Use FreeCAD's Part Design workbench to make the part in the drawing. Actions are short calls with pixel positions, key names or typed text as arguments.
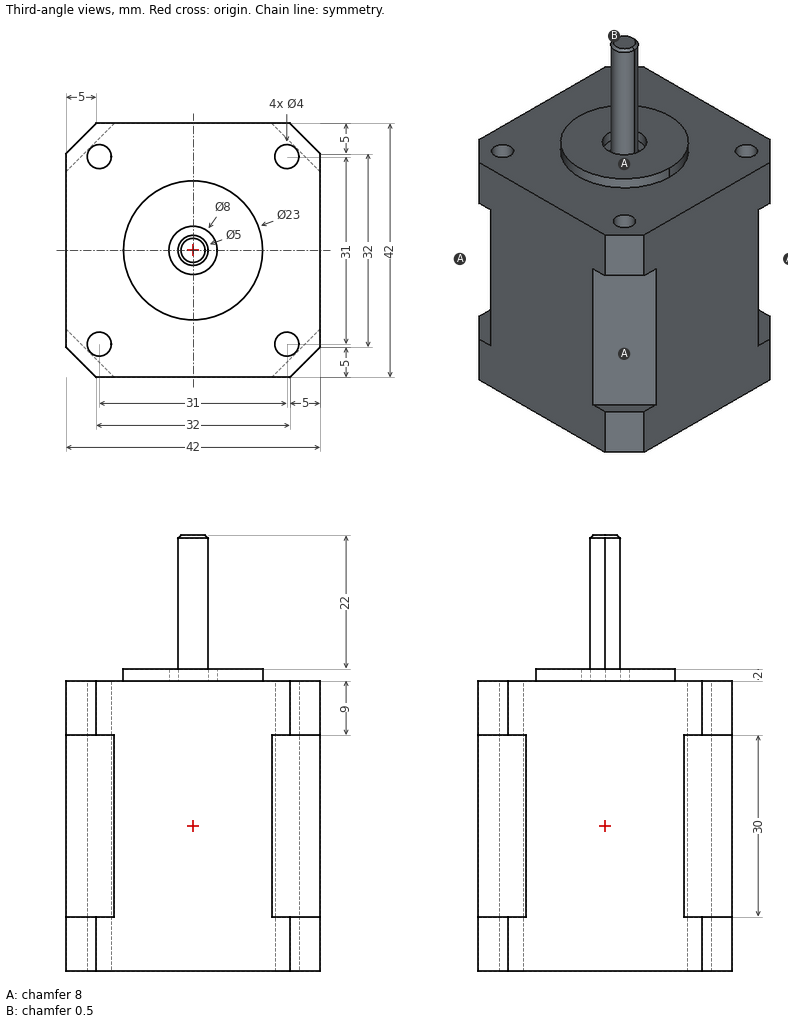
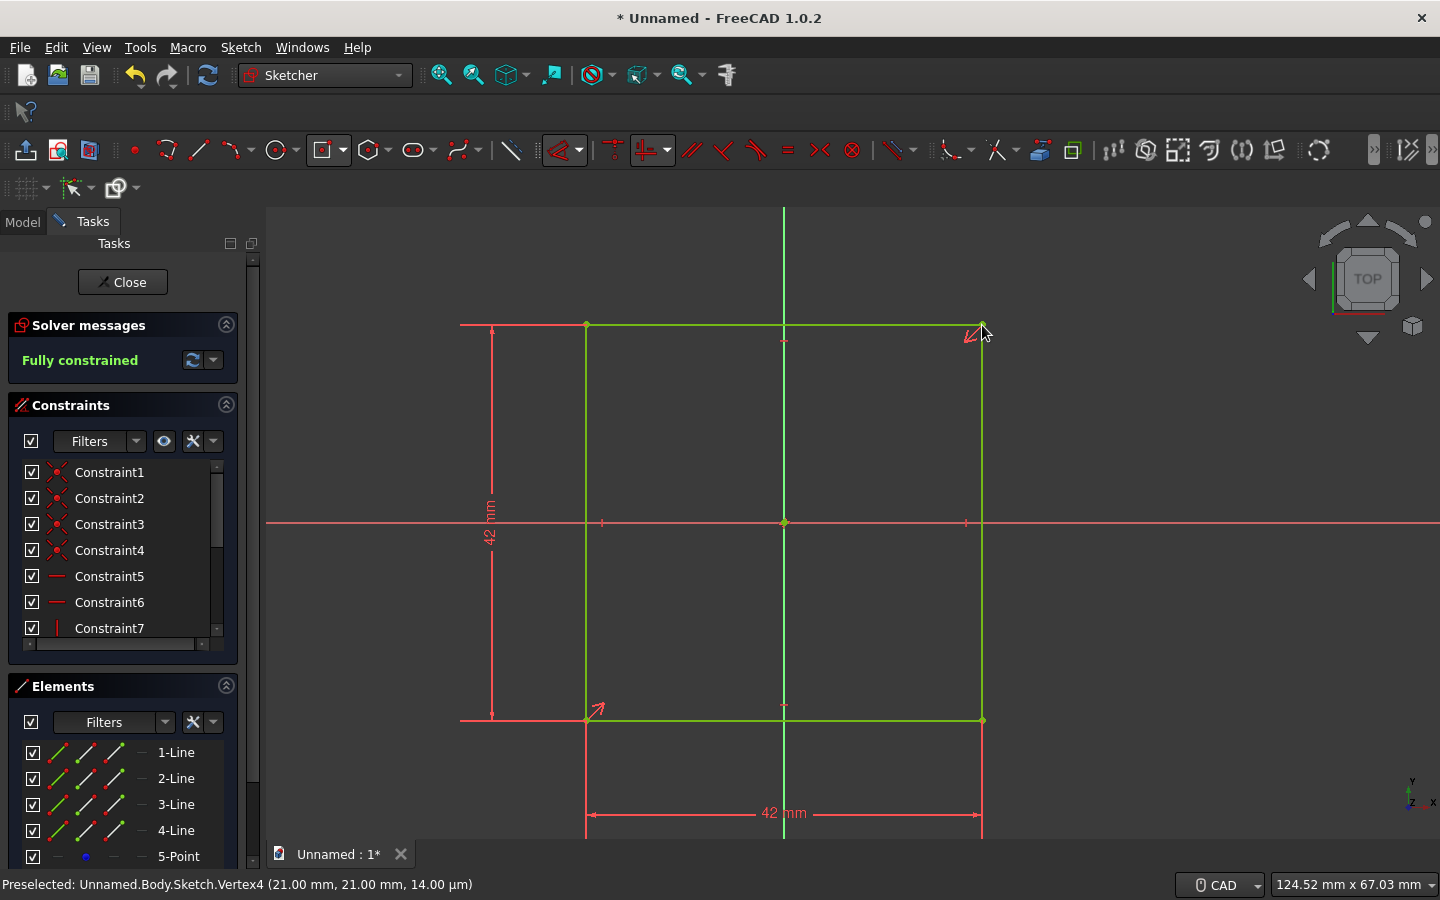
click(123, 282)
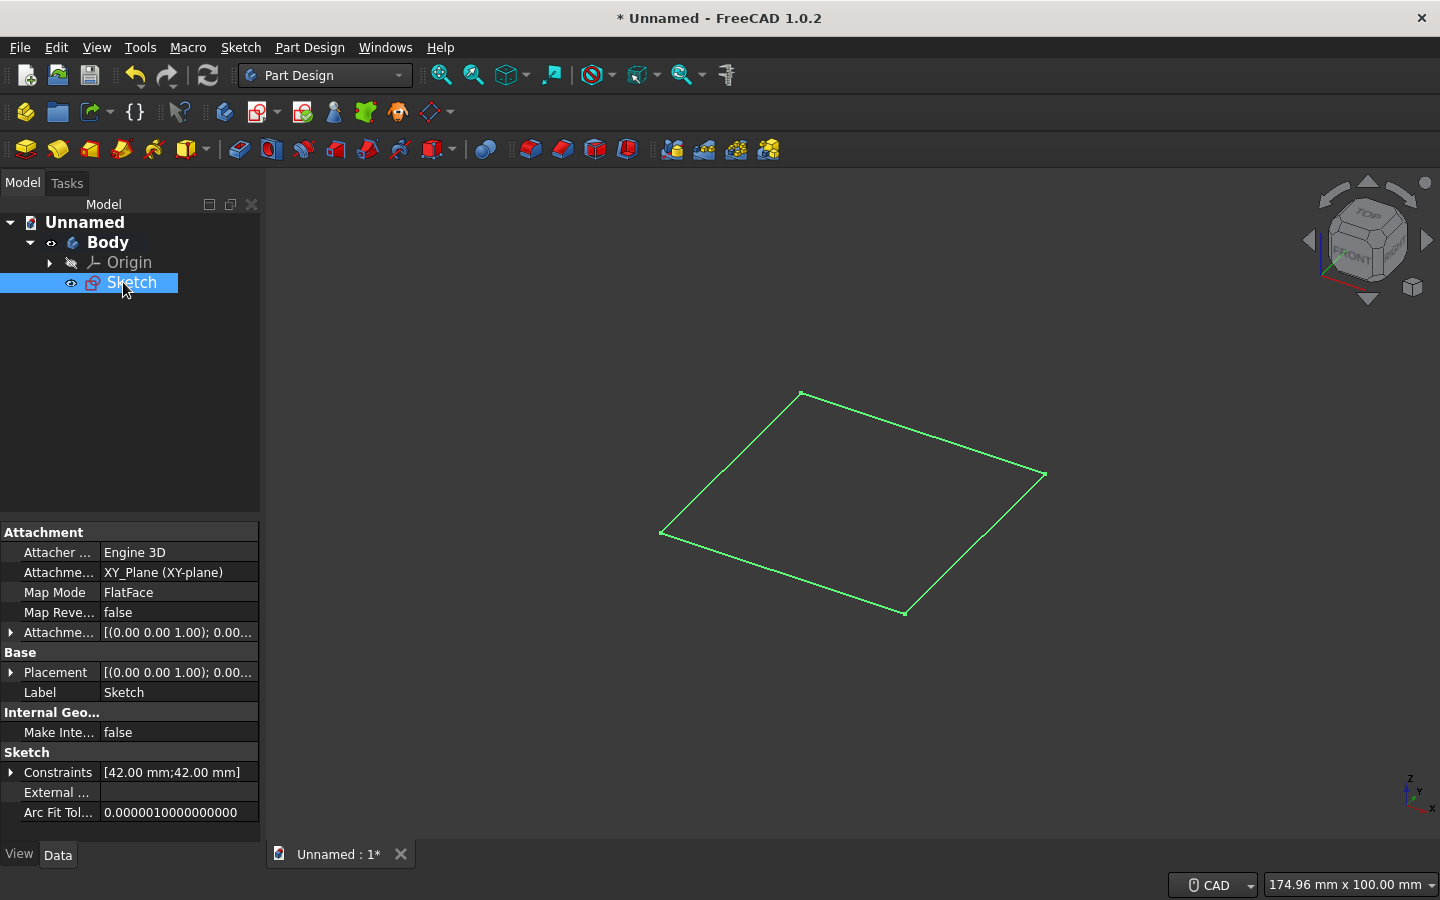
click(26, 150)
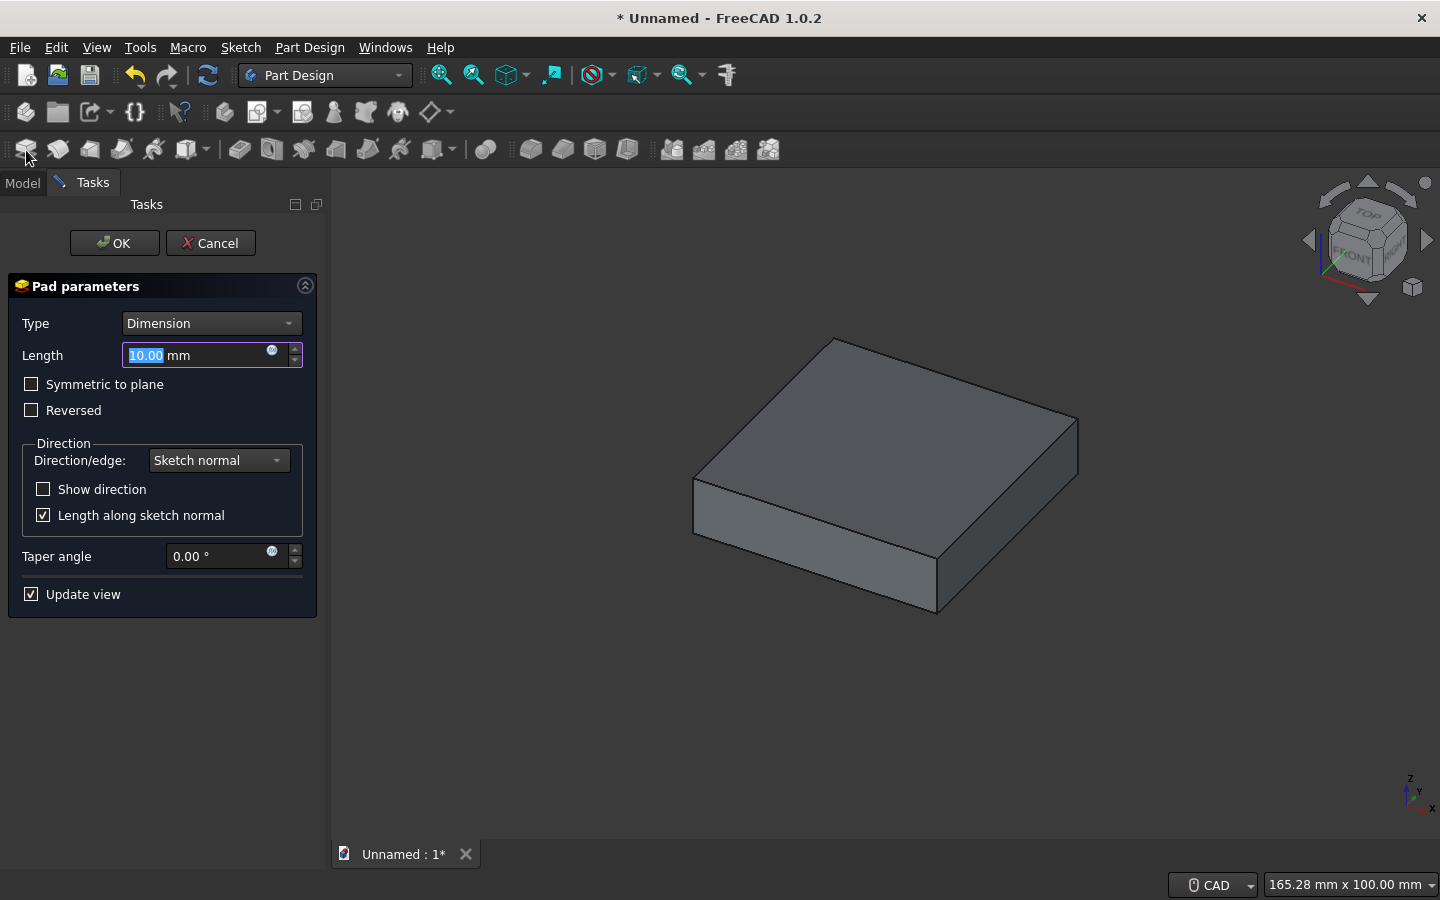
text(30)
key(Tab)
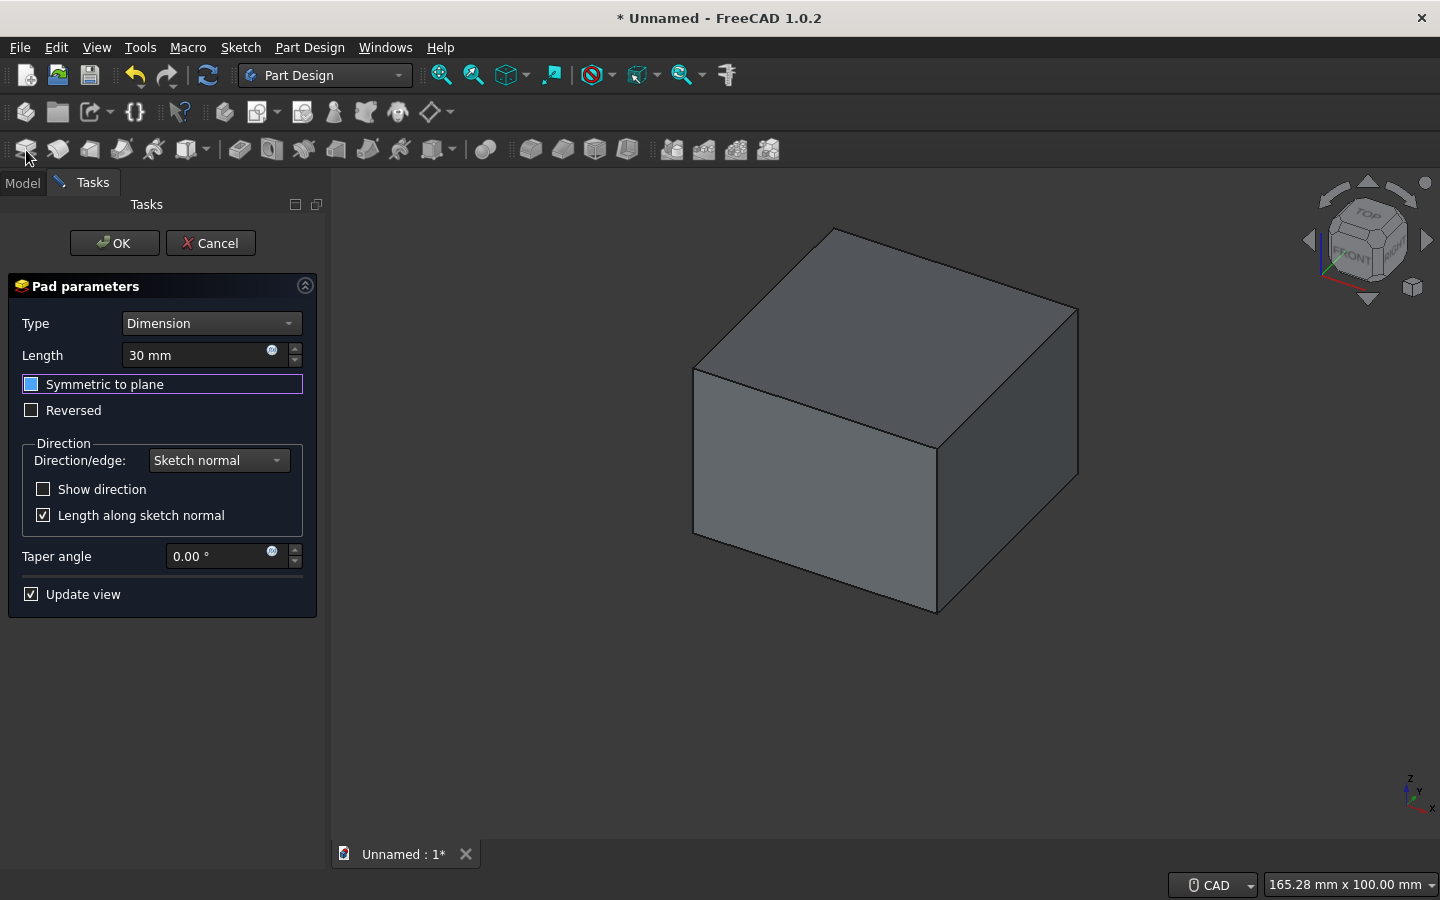
click(30, 384)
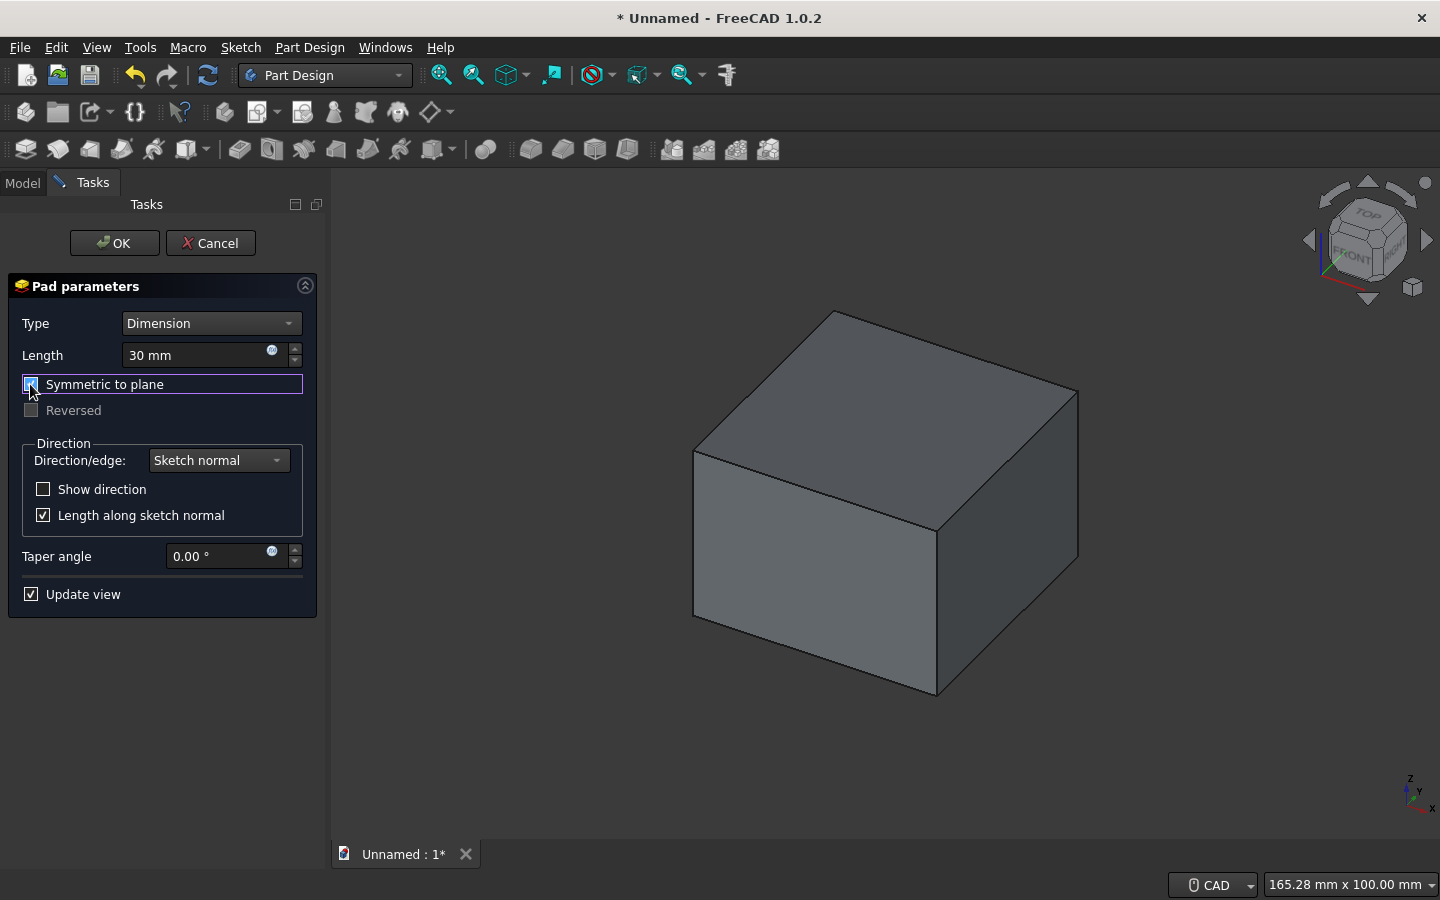
click(115, 243)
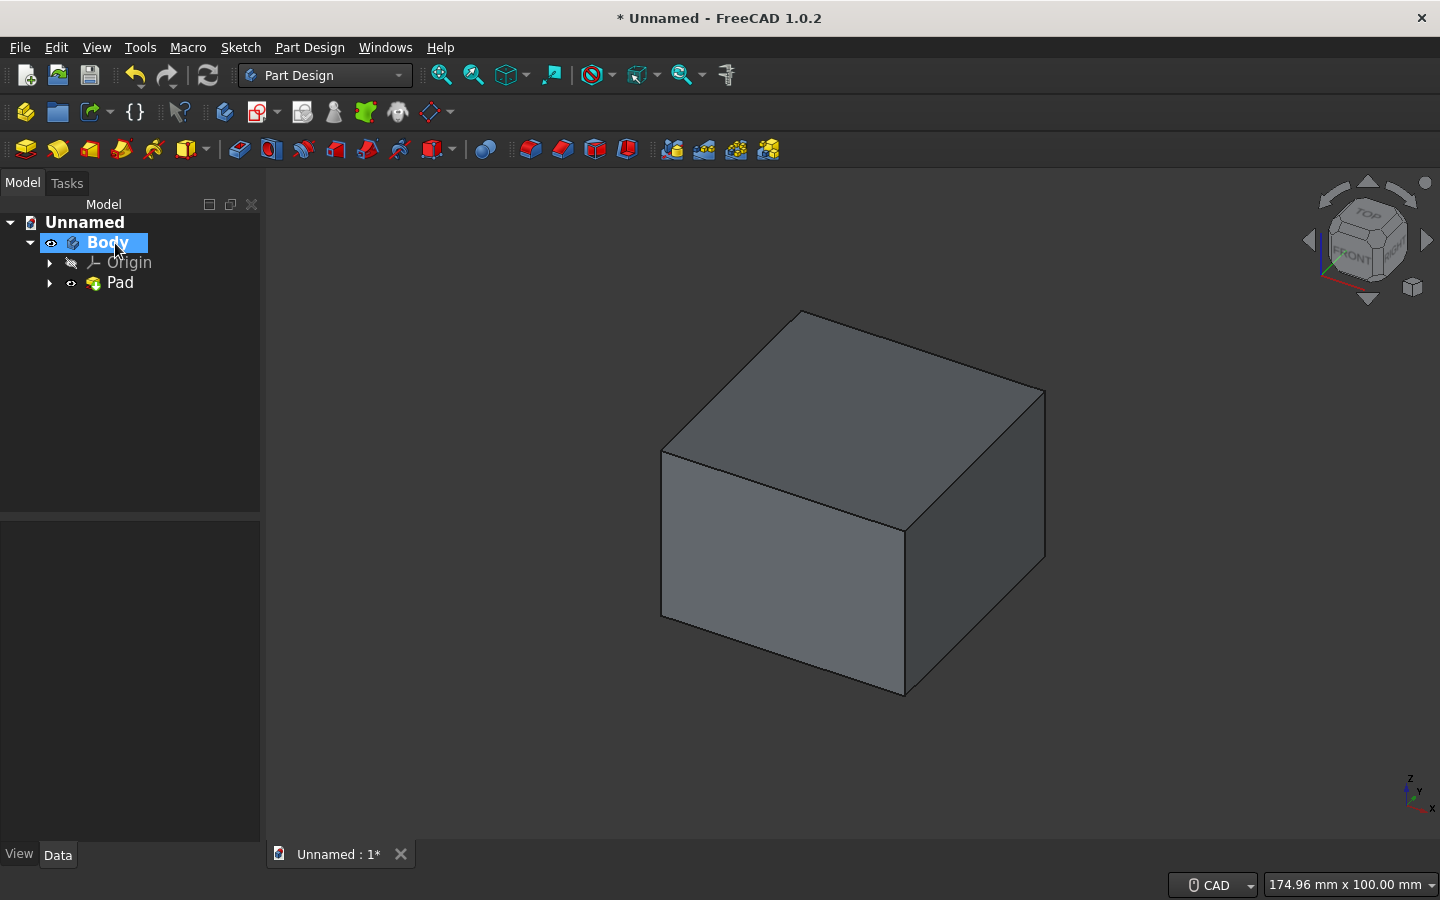
click(905, 613)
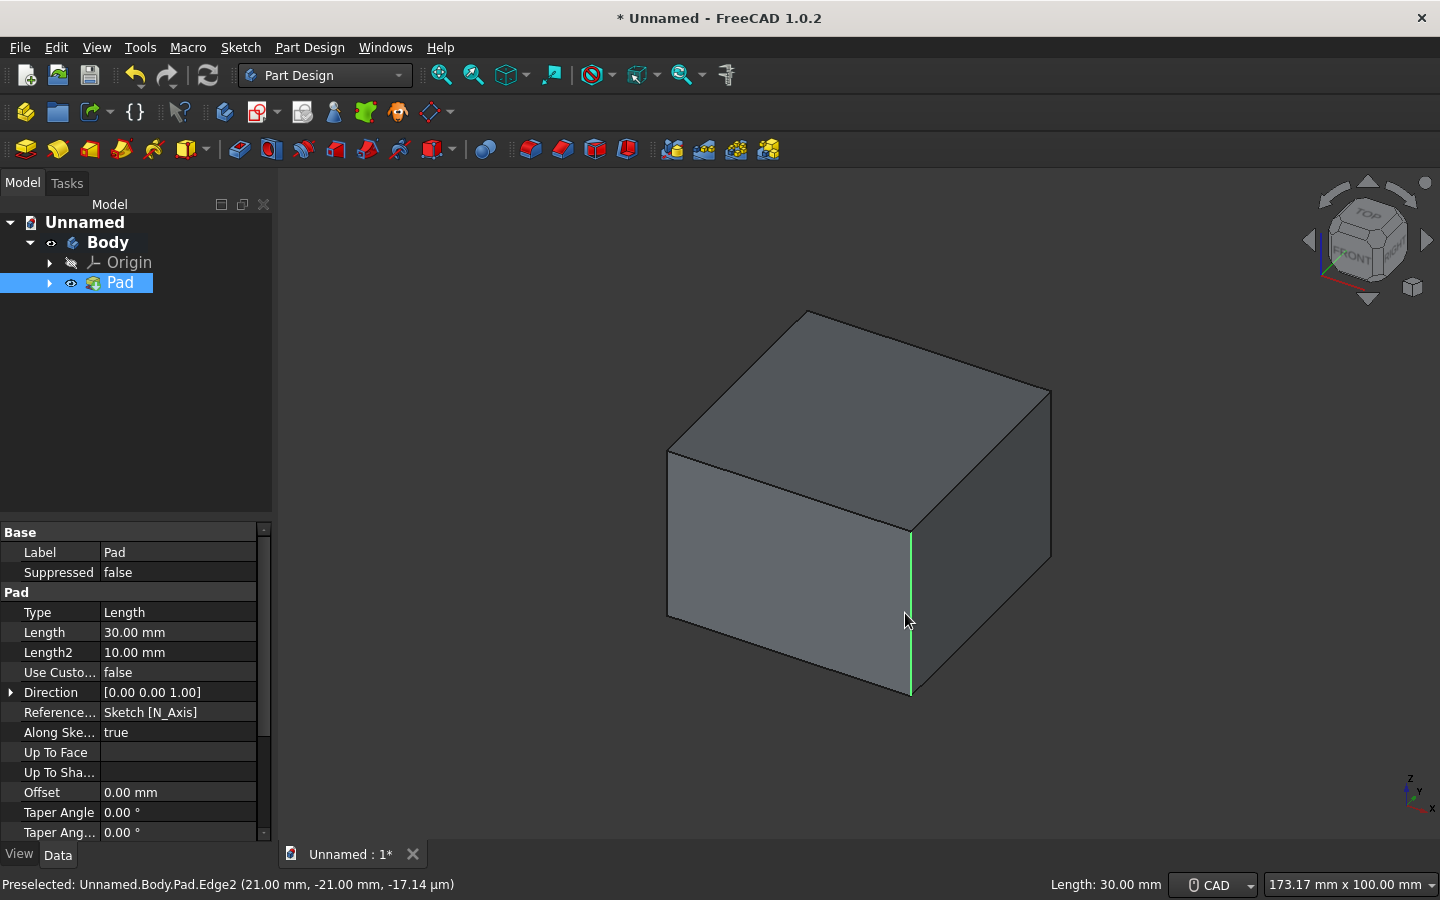
key(0)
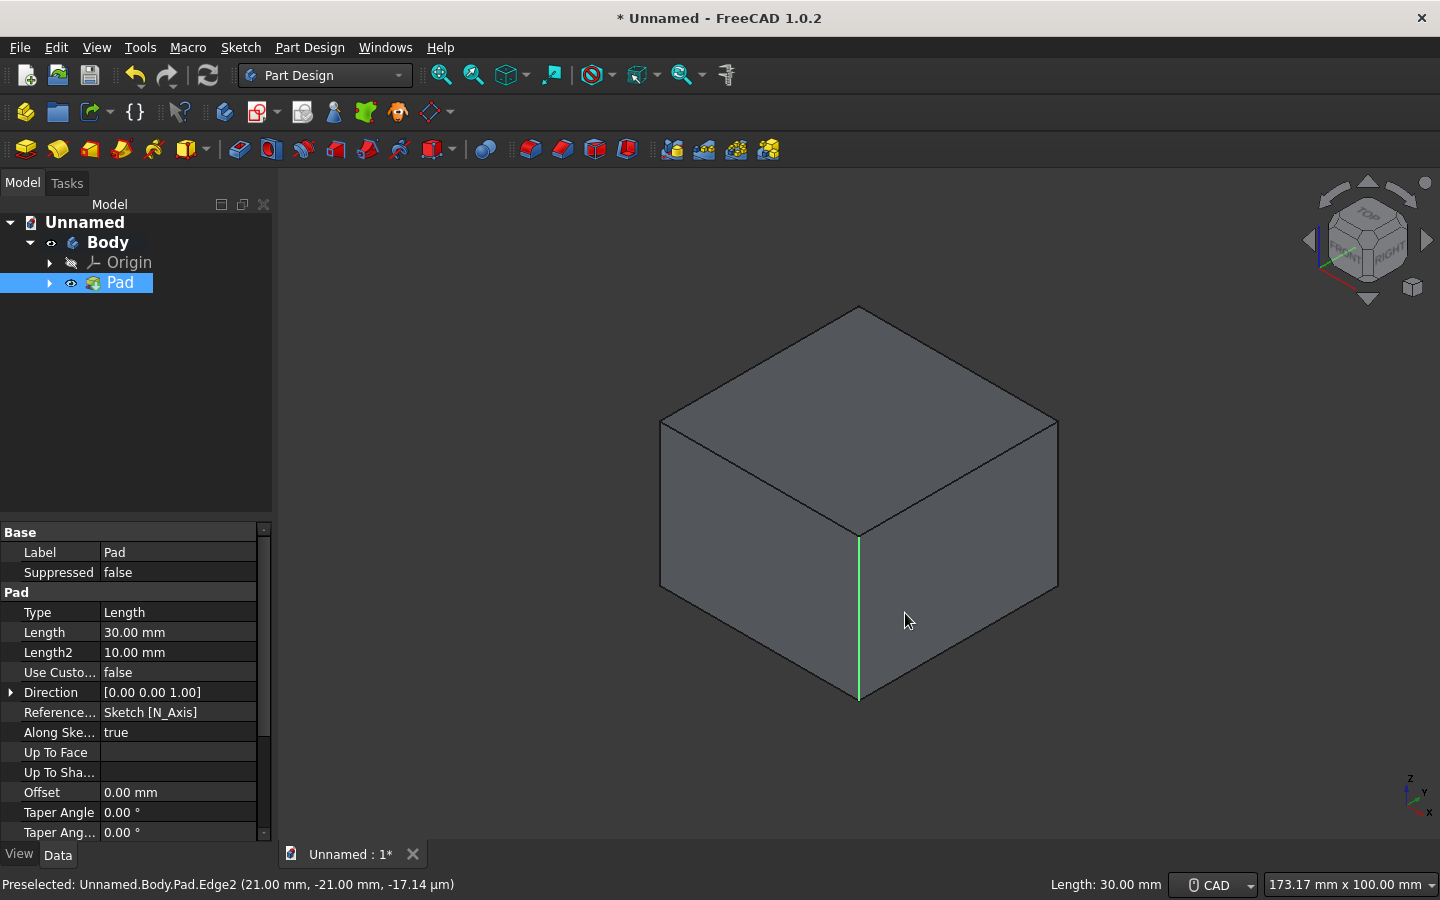
key(2)